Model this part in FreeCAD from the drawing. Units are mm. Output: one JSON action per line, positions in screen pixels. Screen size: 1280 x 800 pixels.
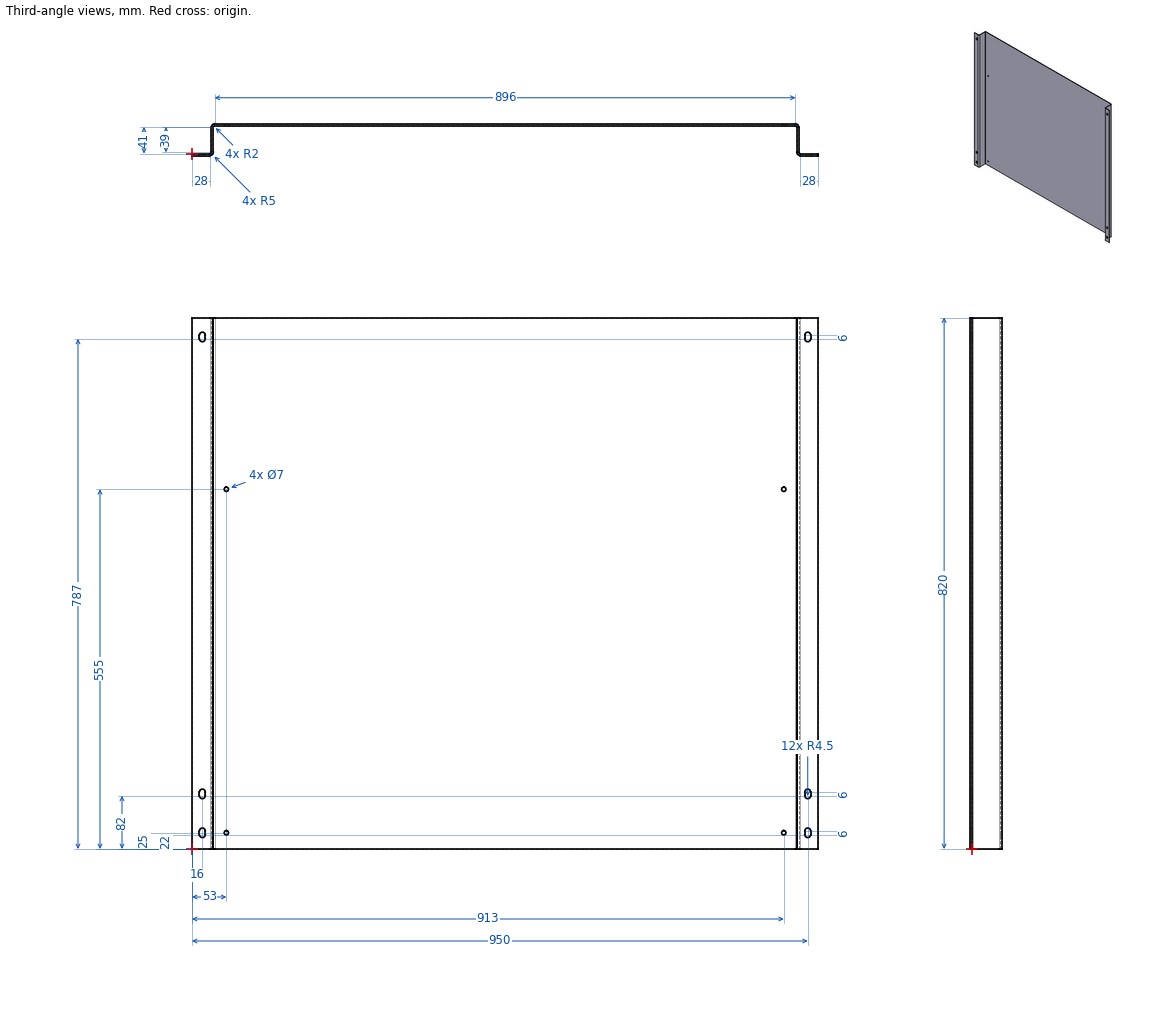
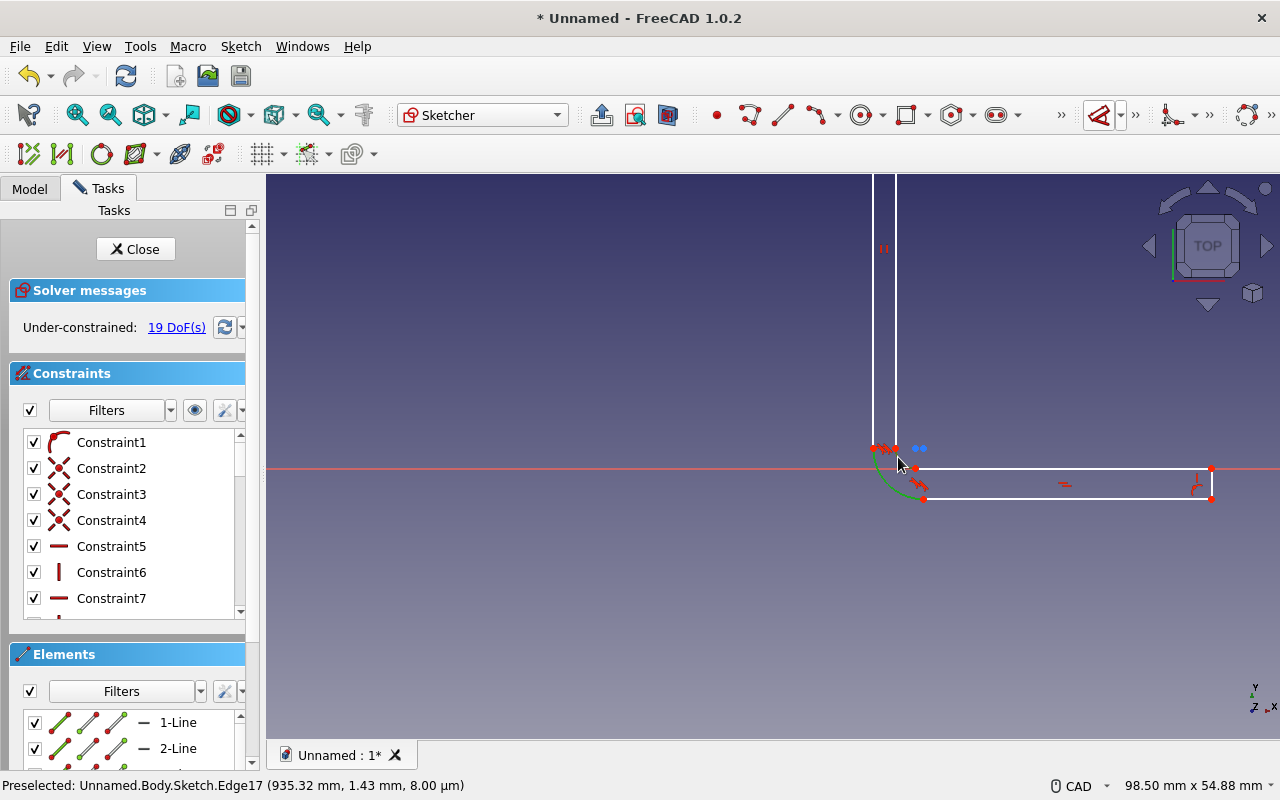
{"action": "key", "text": "c"}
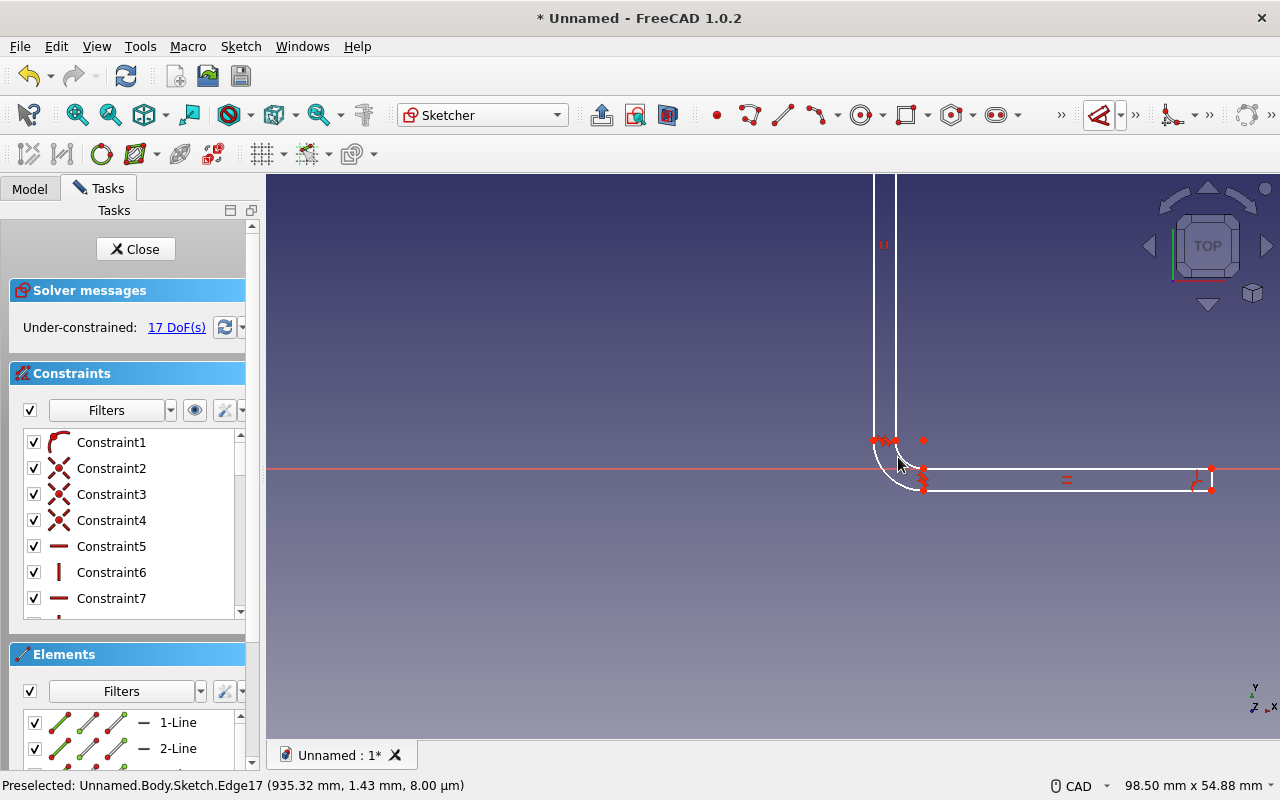
{"action": "scroll", "coordinate": [994, 470], "scroll_direction": "down", "scroll_amount": 14}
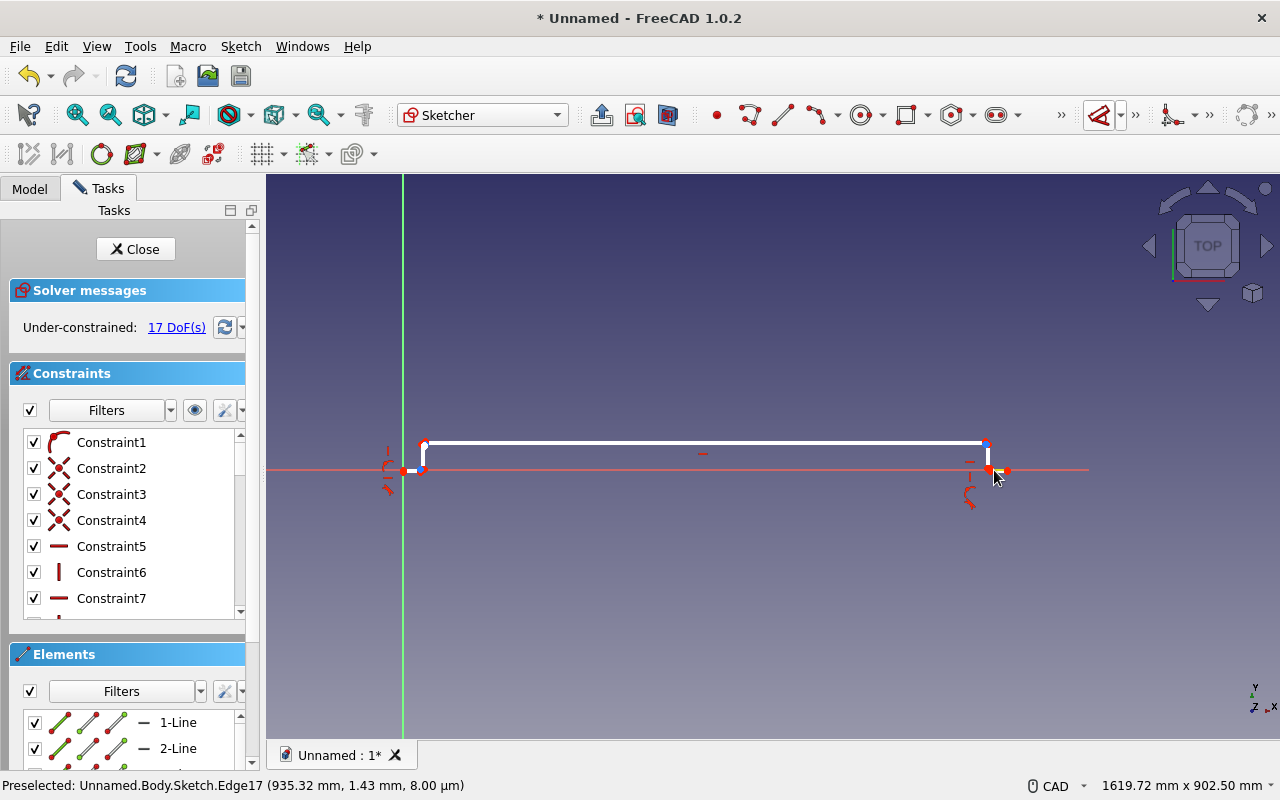
{"action": "scroll", "coordinate": [987, 444], "scroll_direction": "up", "scroll_amount": 14}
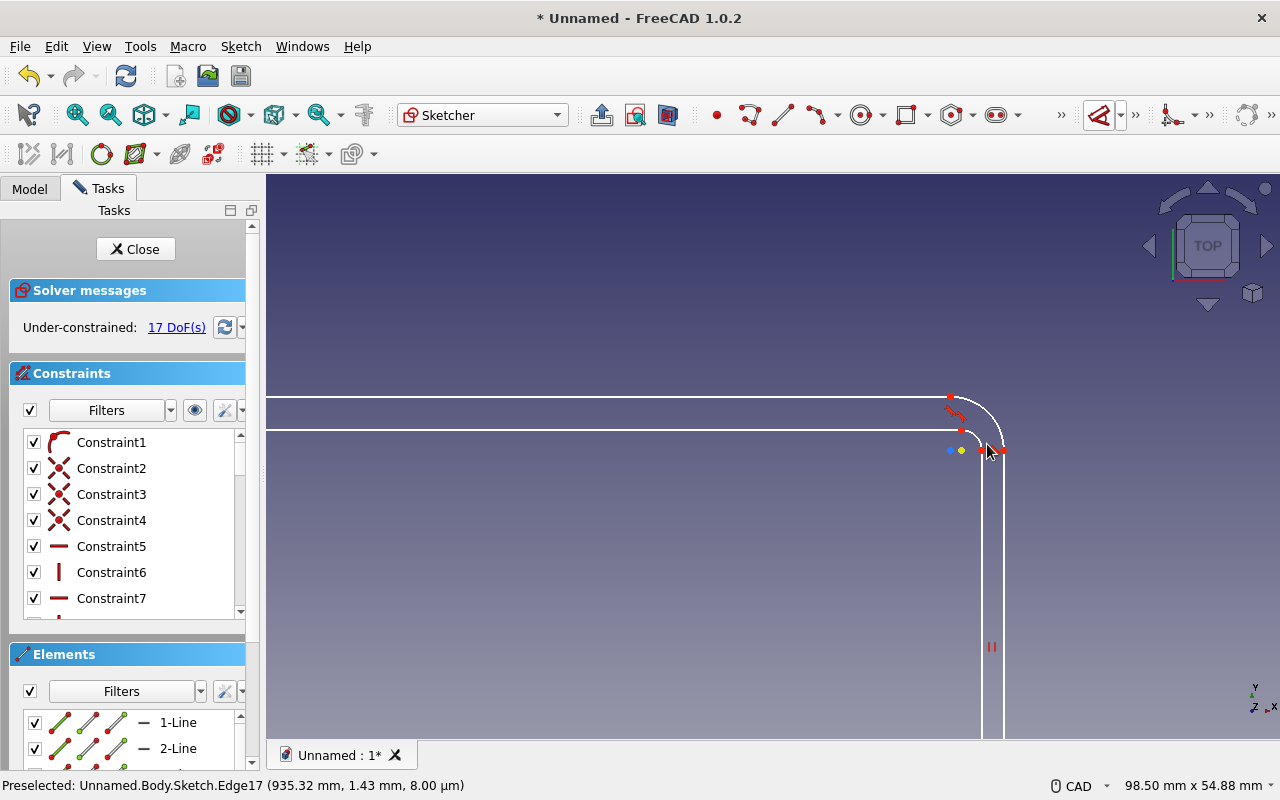
{"action": "left_click", "coordinate": [980, 441]}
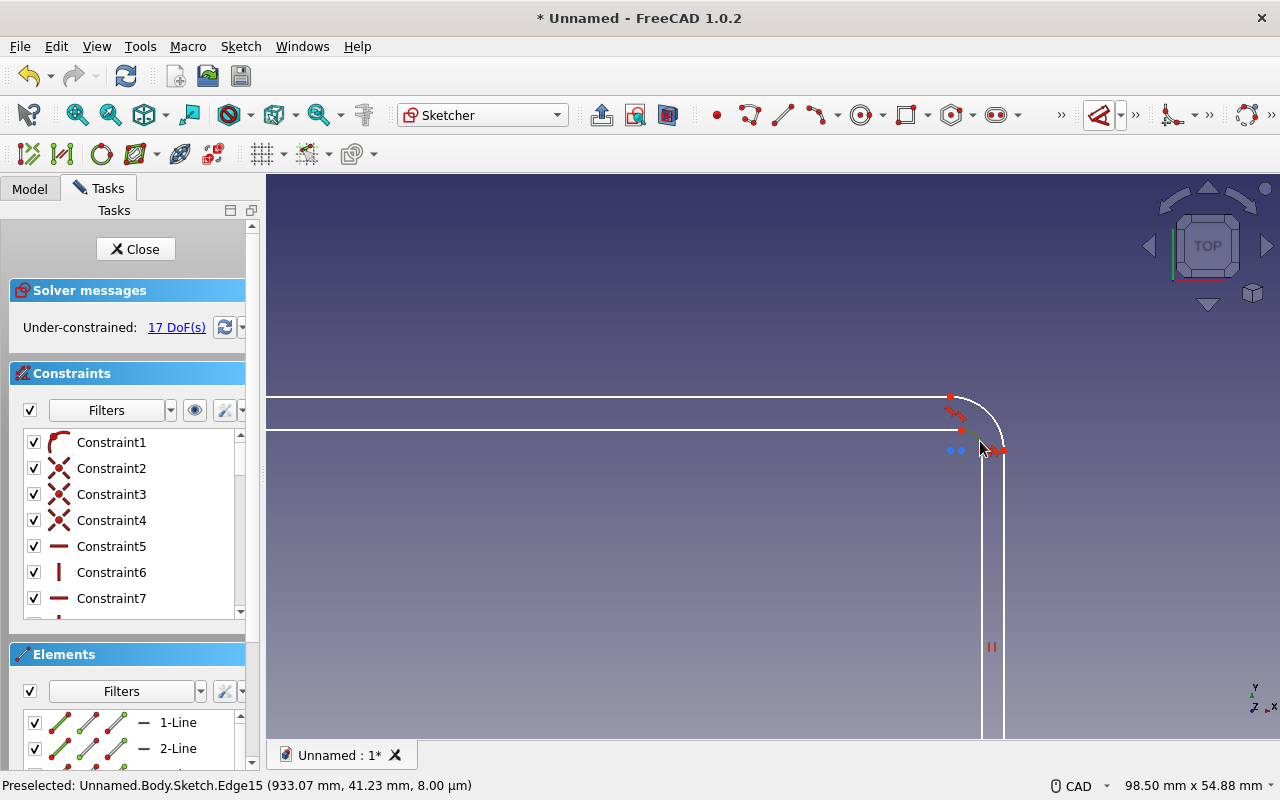
{"action": "left_click", "coordinate": [998, 426]}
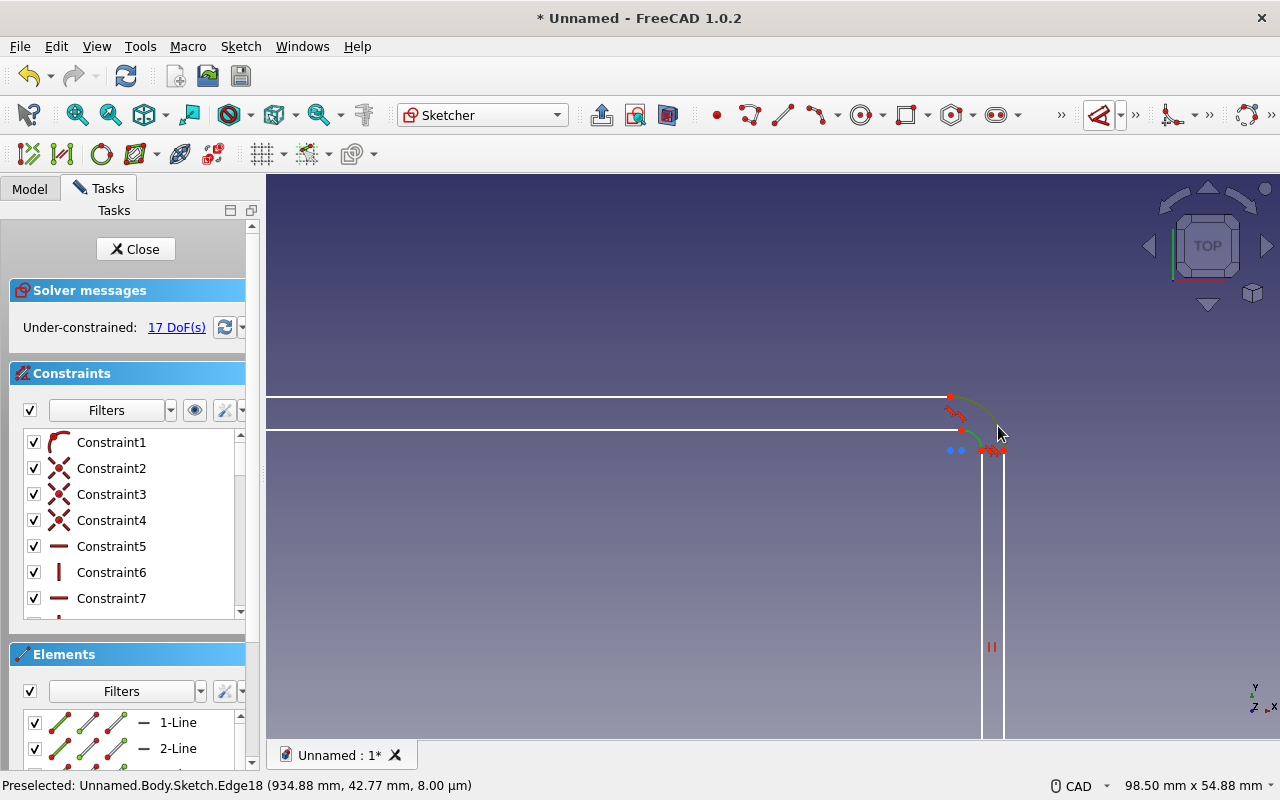
{"action": "key", "text": "c"}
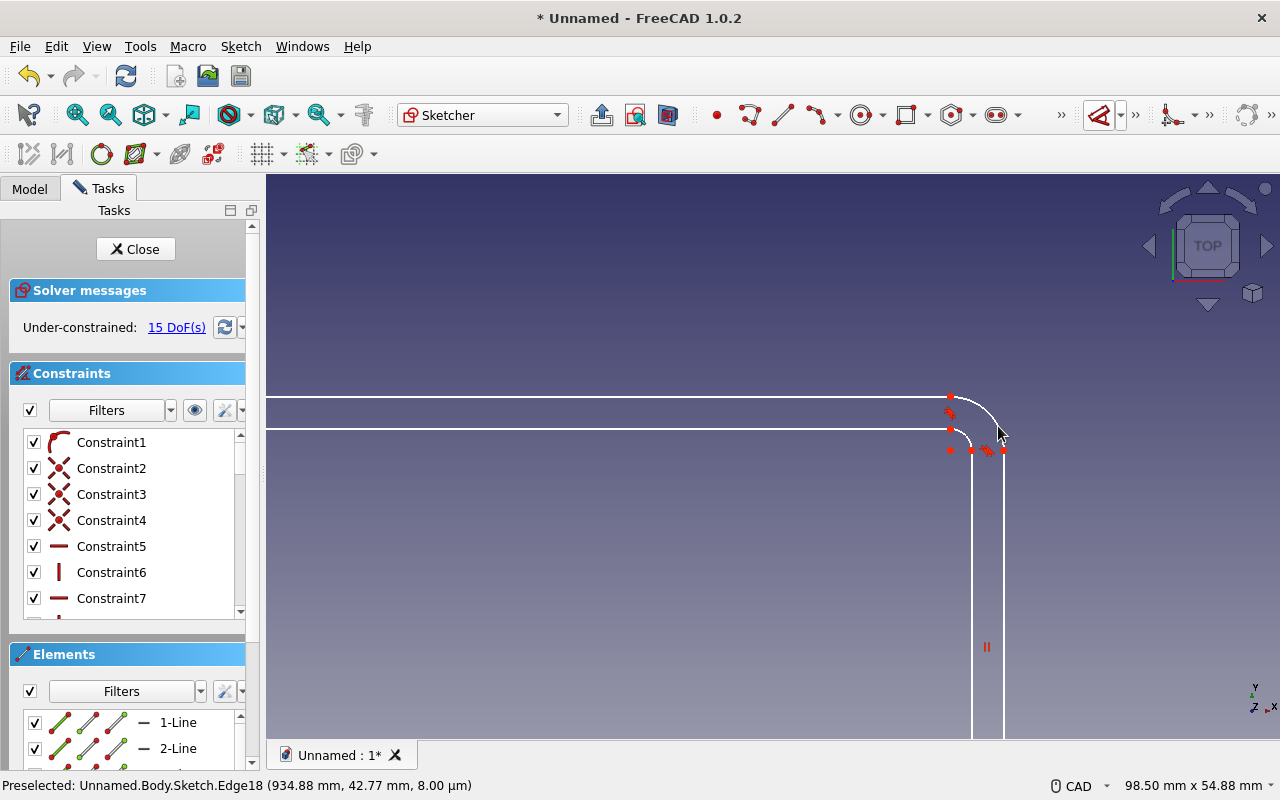
{"action": "scroll", "coordinate": [987, 444], "scroll_direction": "down", "scroll_amount": 14}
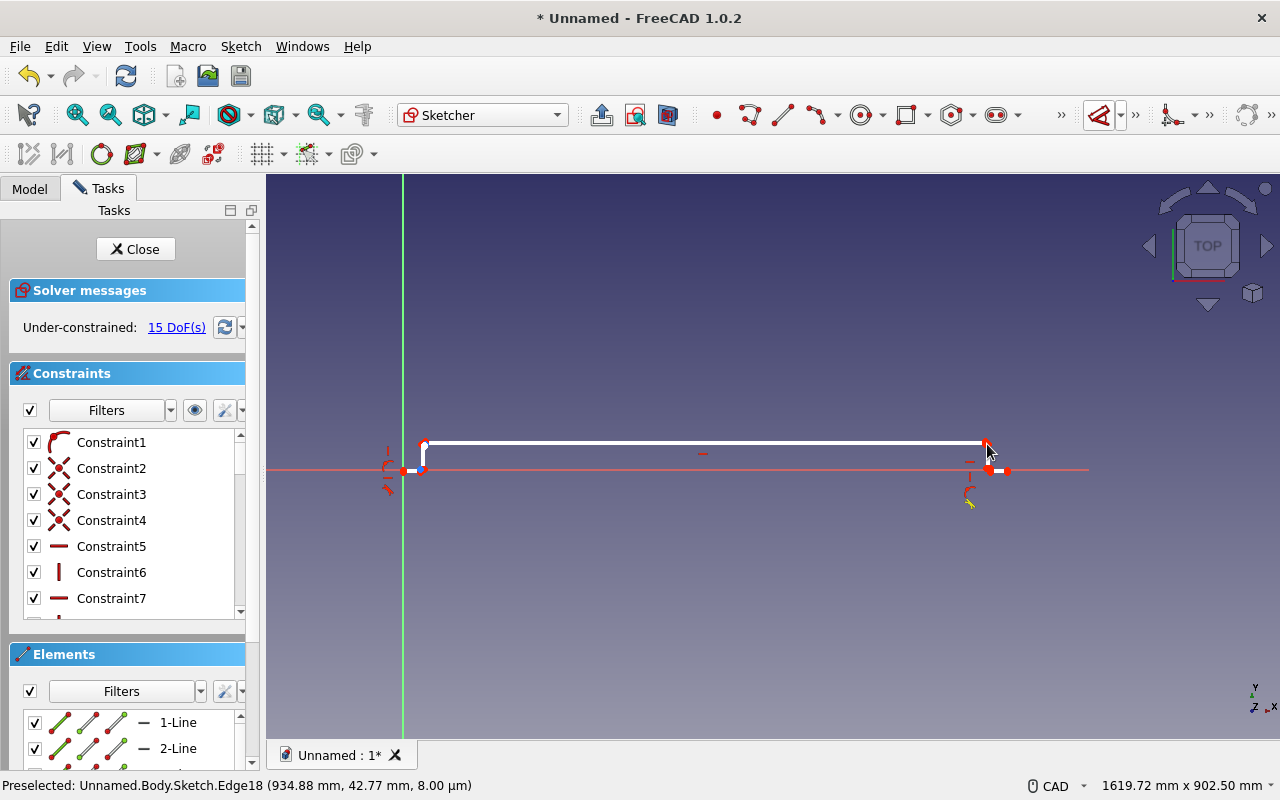
{"action": "scroll", "coordinate": [424, 444], "scroll_direction": "up", "scroll_amount": 14}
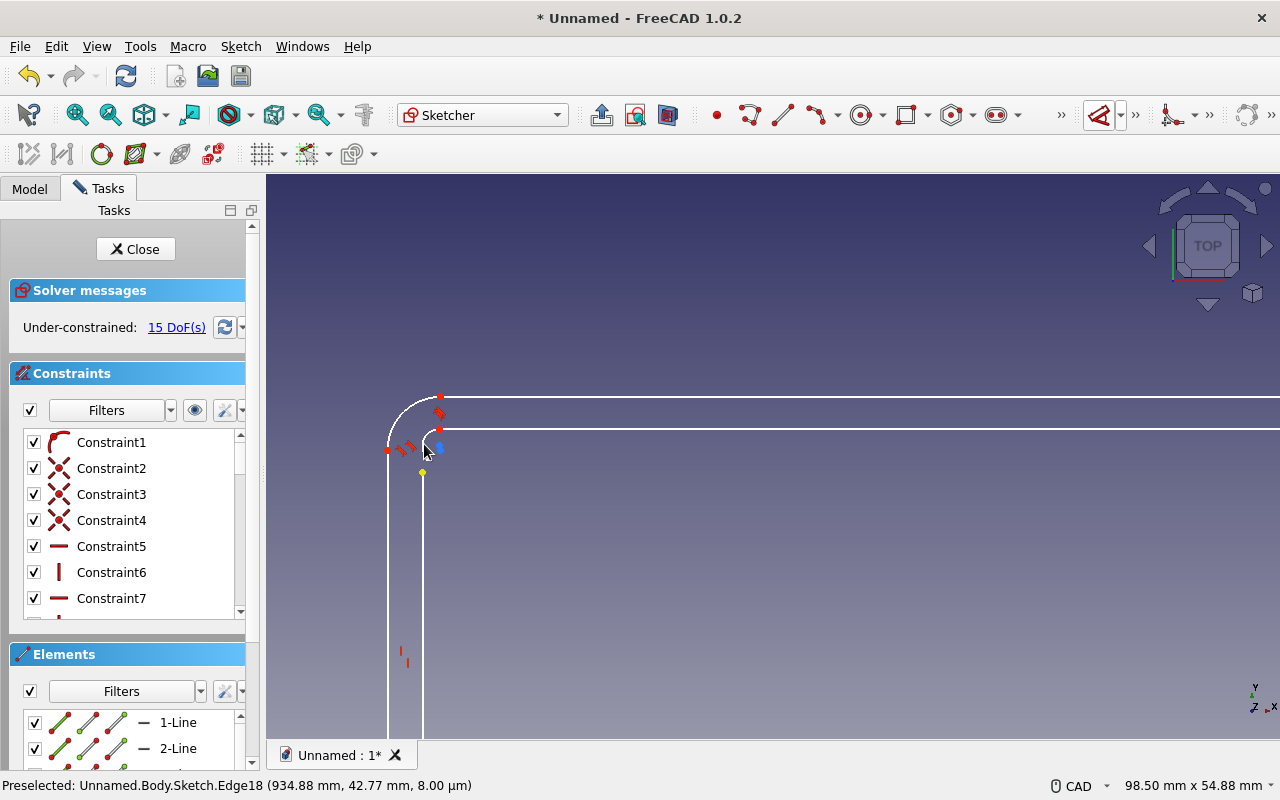
{"action": "left_click", "coordinate": [428, 433]}